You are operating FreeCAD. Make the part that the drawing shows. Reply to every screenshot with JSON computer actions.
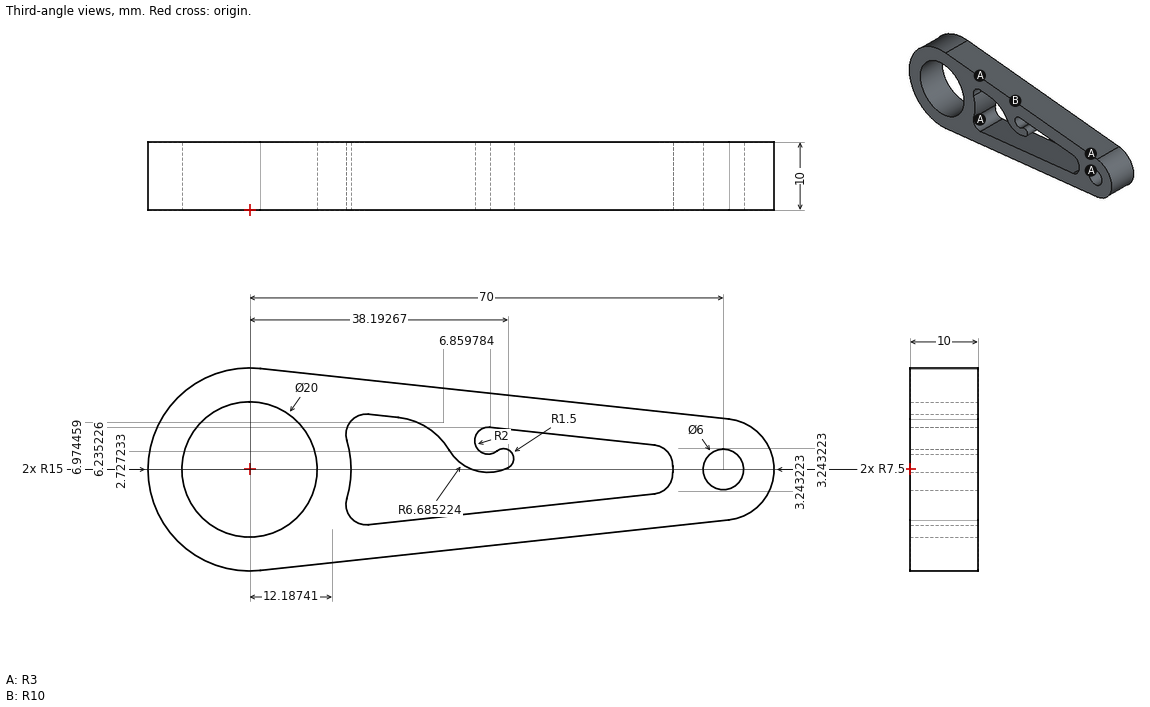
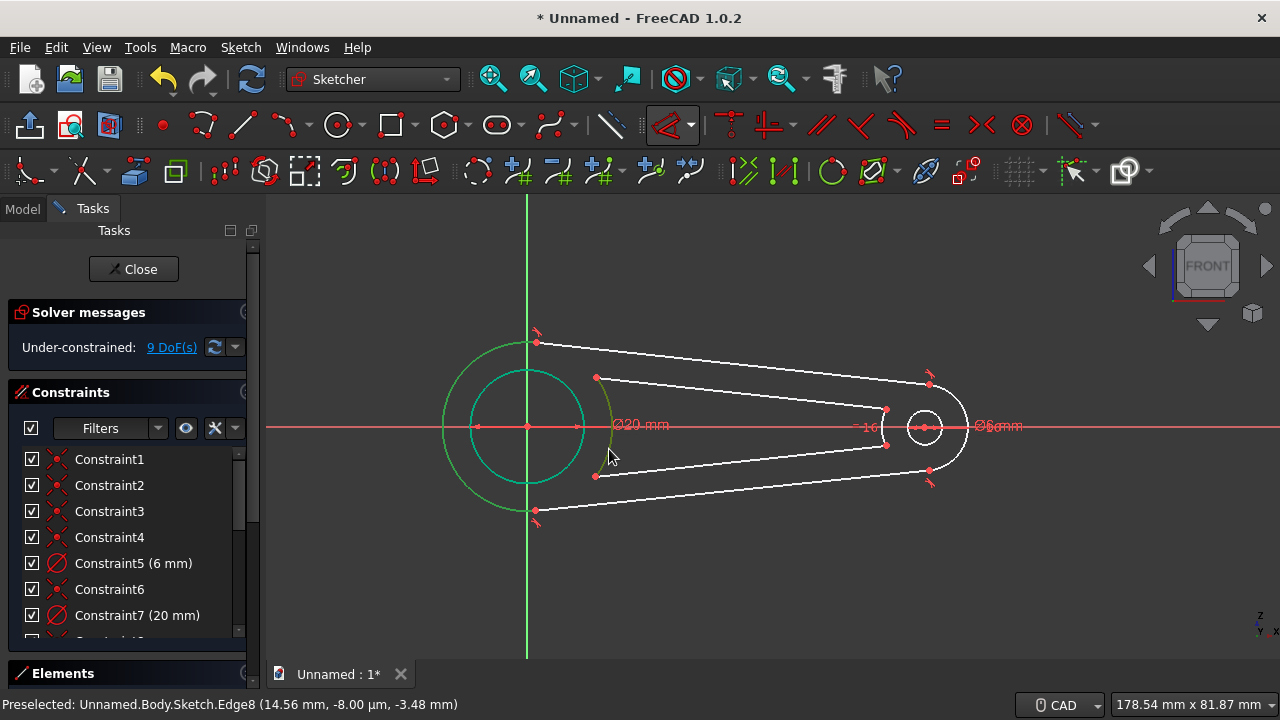
{"action": "left_click", "coordinate": [942, 126]}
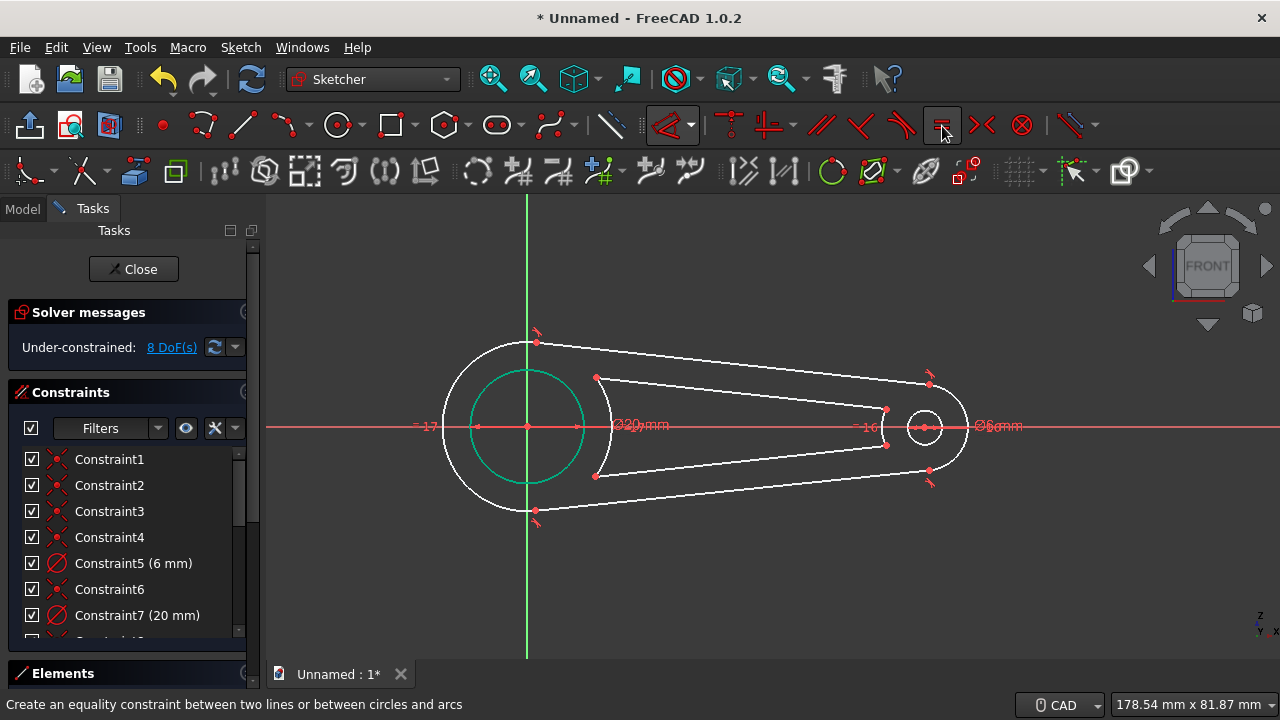
{"action": "left_click", "coordinate": [925, 428]}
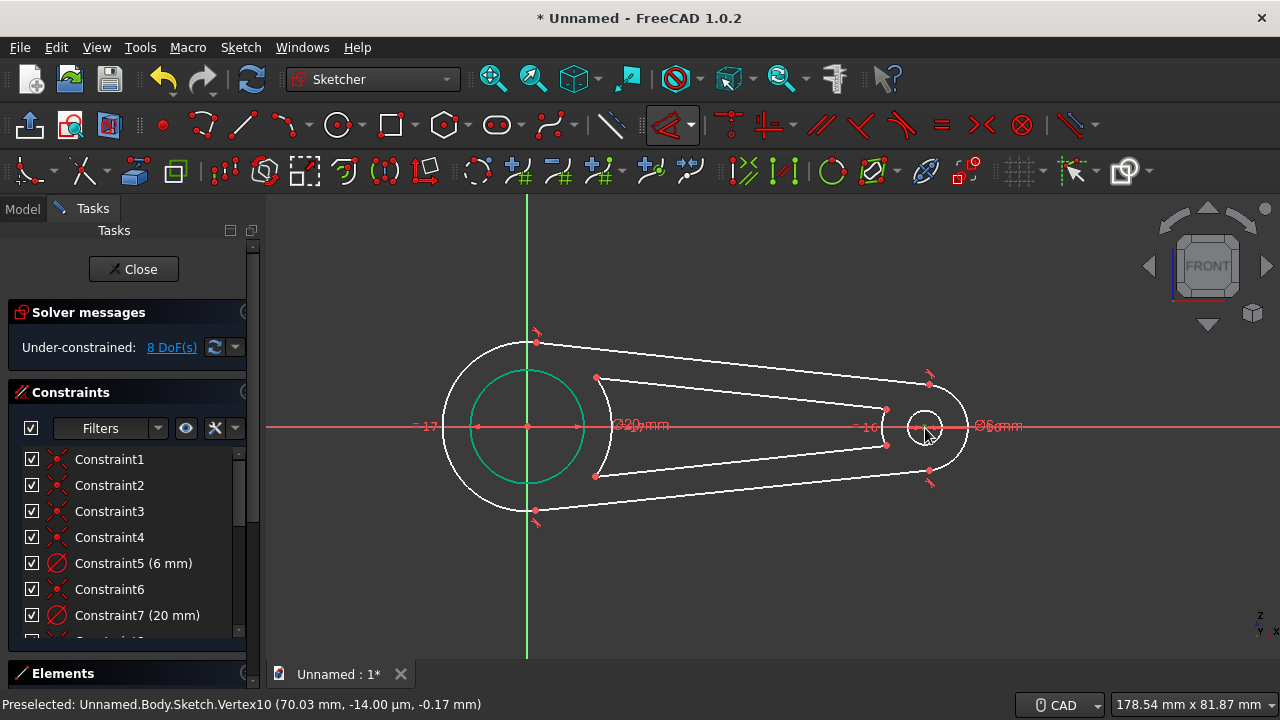
{"action": "left_click", "coordinate": [353, 427]}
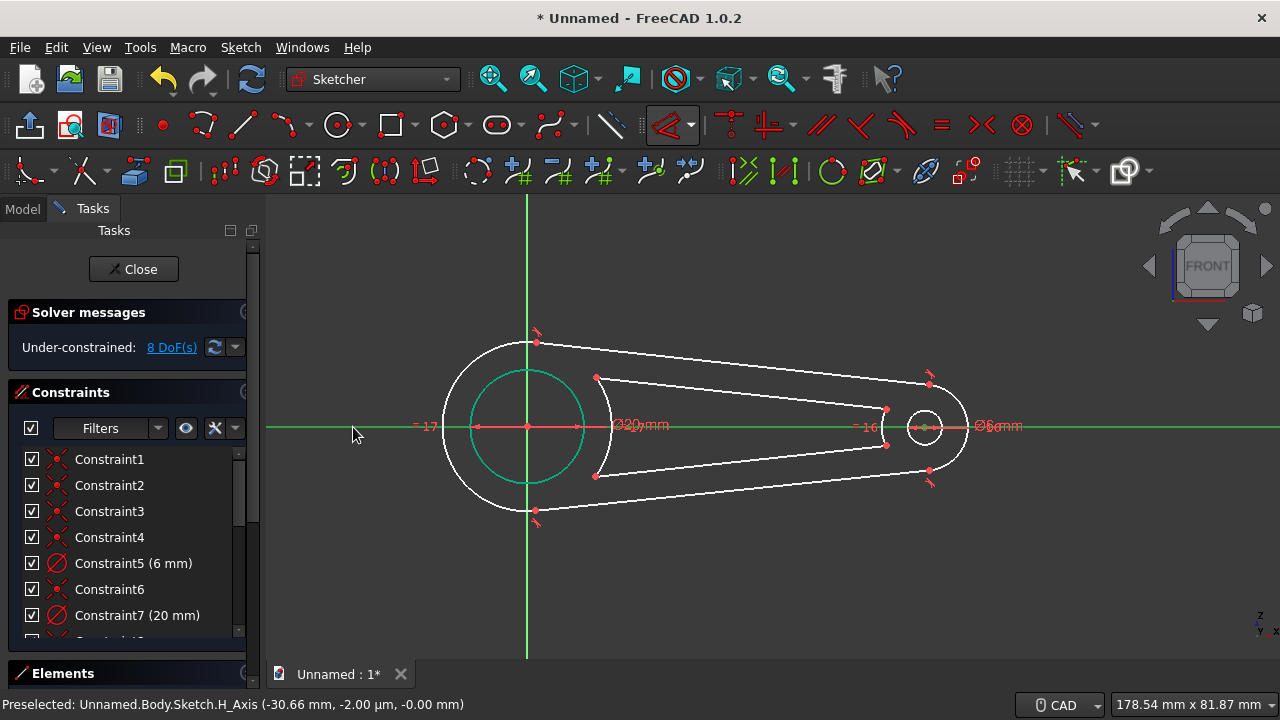
{"action": "left_click", "coordinate": [730, 126]}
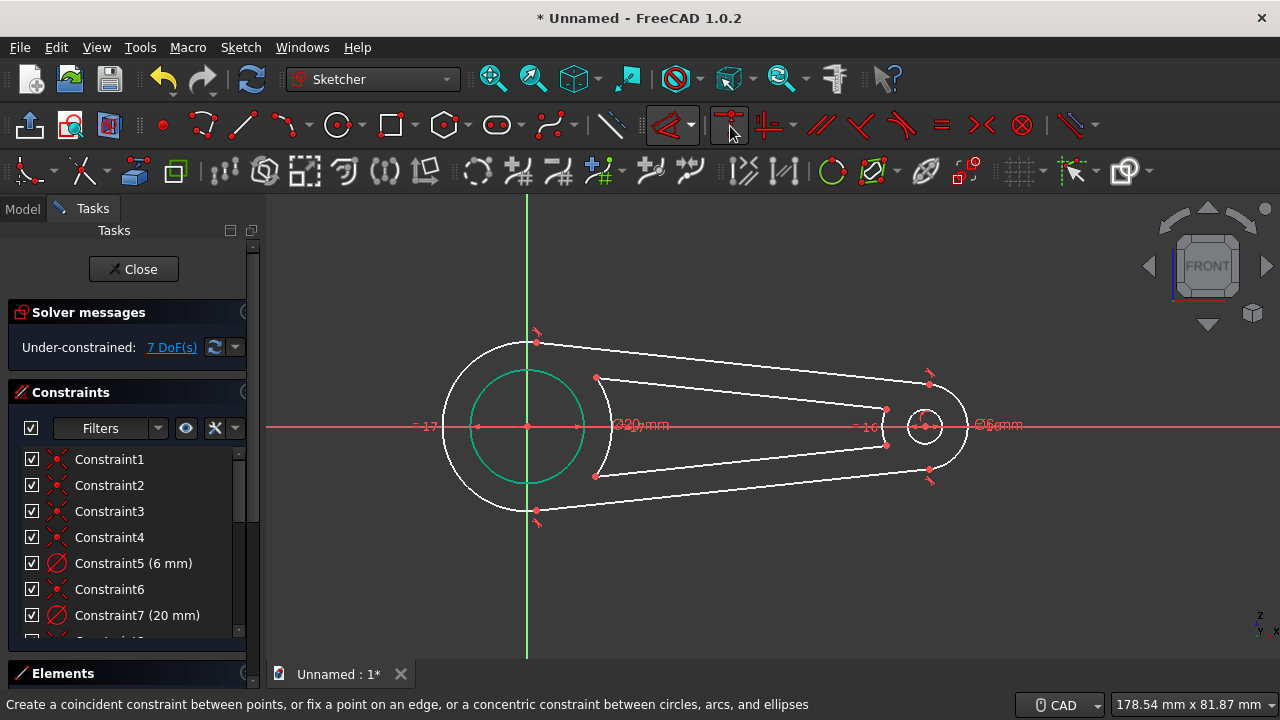
{"action": "left_click", "coordinate": [666, 126]}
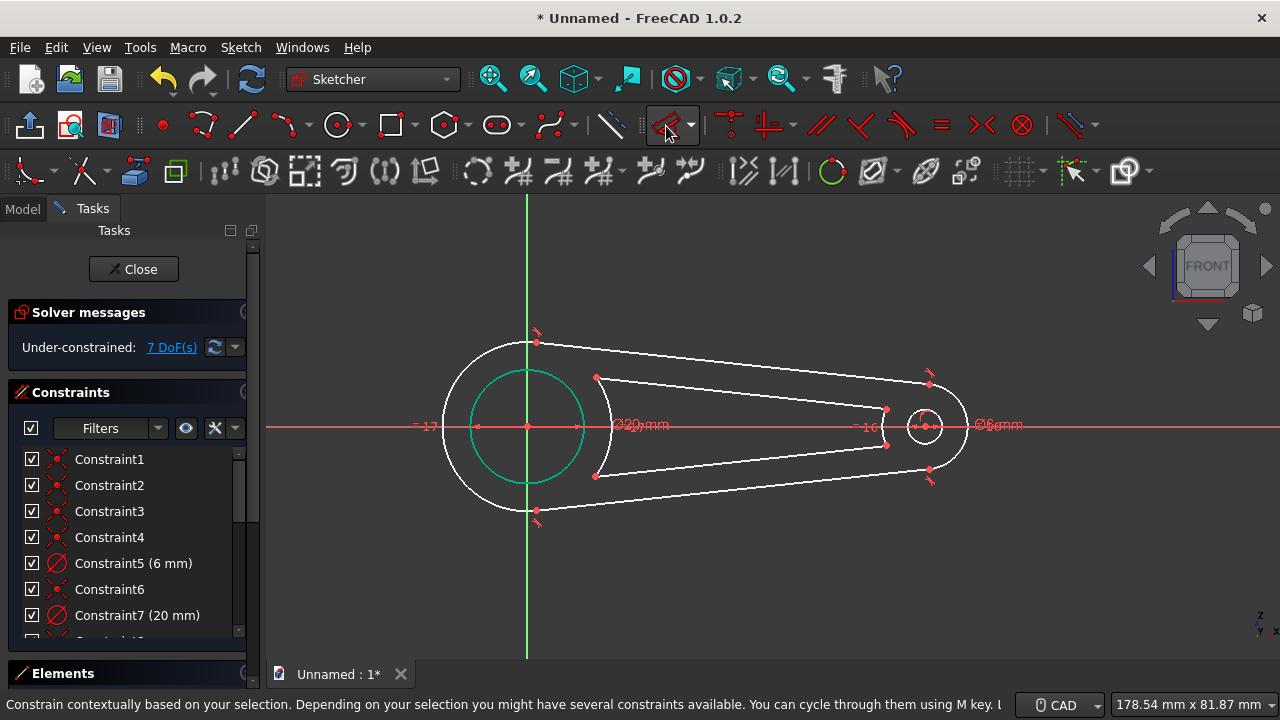
{"action": "left_click", "coordinate": [461, 374]}
{"action": "left_click", "coordinate": [436, 354]}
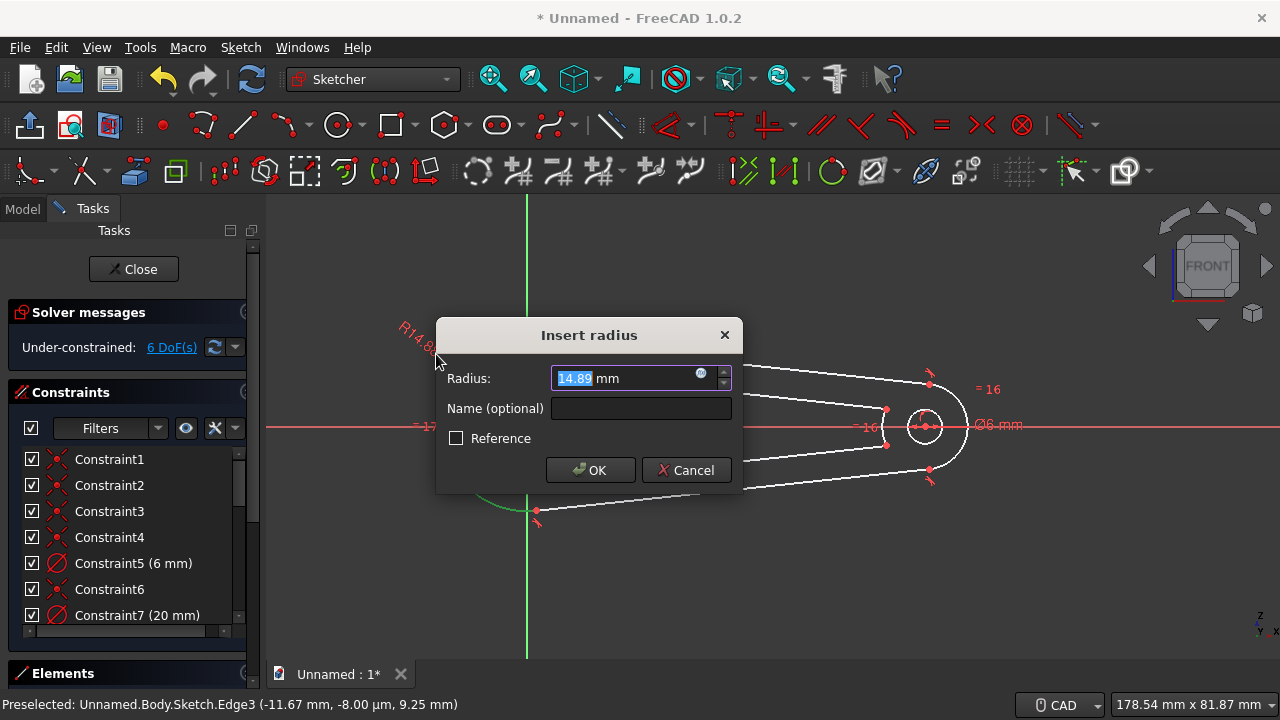
{"action": "type", "text": "15"}
{"action": "key", "text": "Return"}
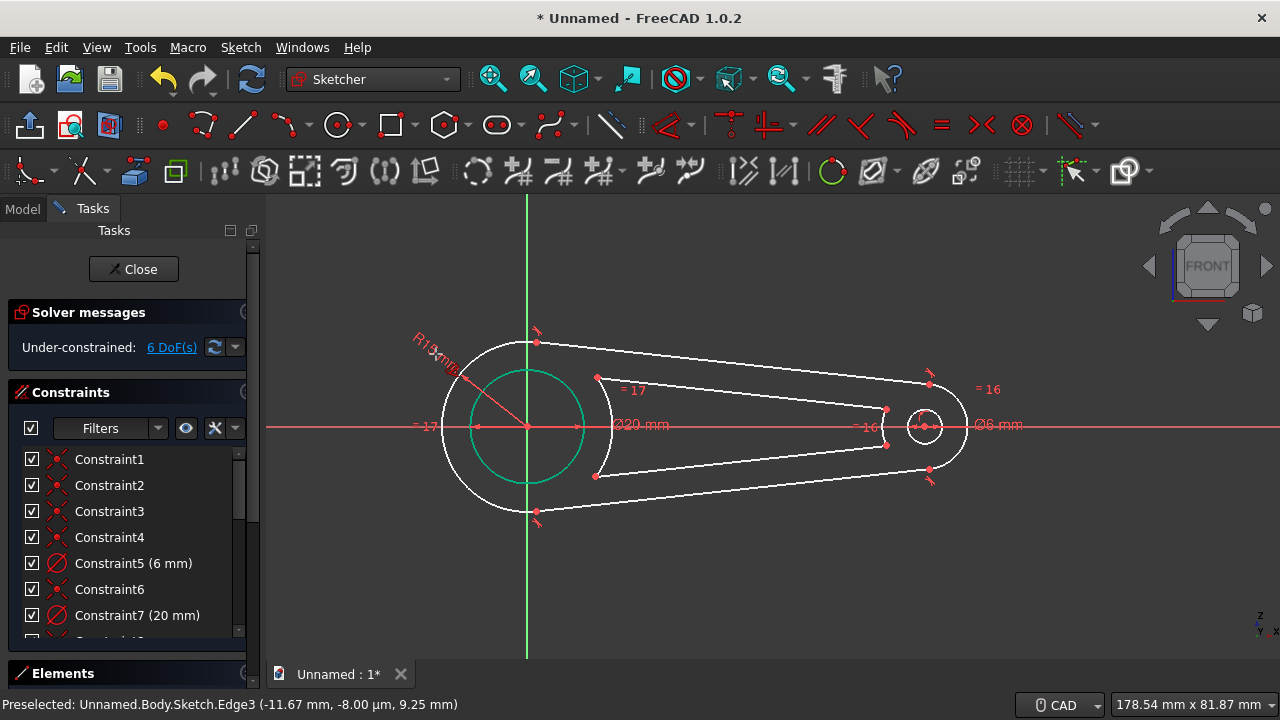
{"action": "left_click", "coordinate": [960, 450]}
{"action": "left_click", "coordinate": [987, 468]}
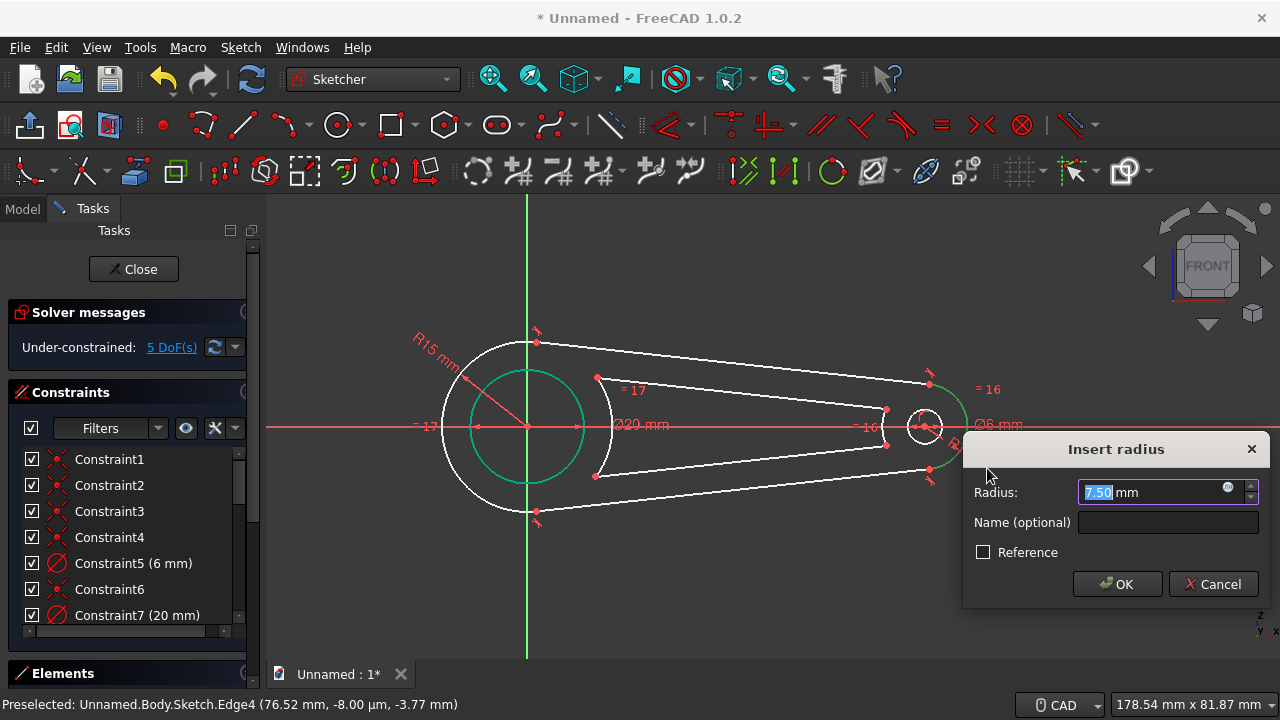
{"action": "type", "text": "7.5"}
{"action": "key", "text": "Return"}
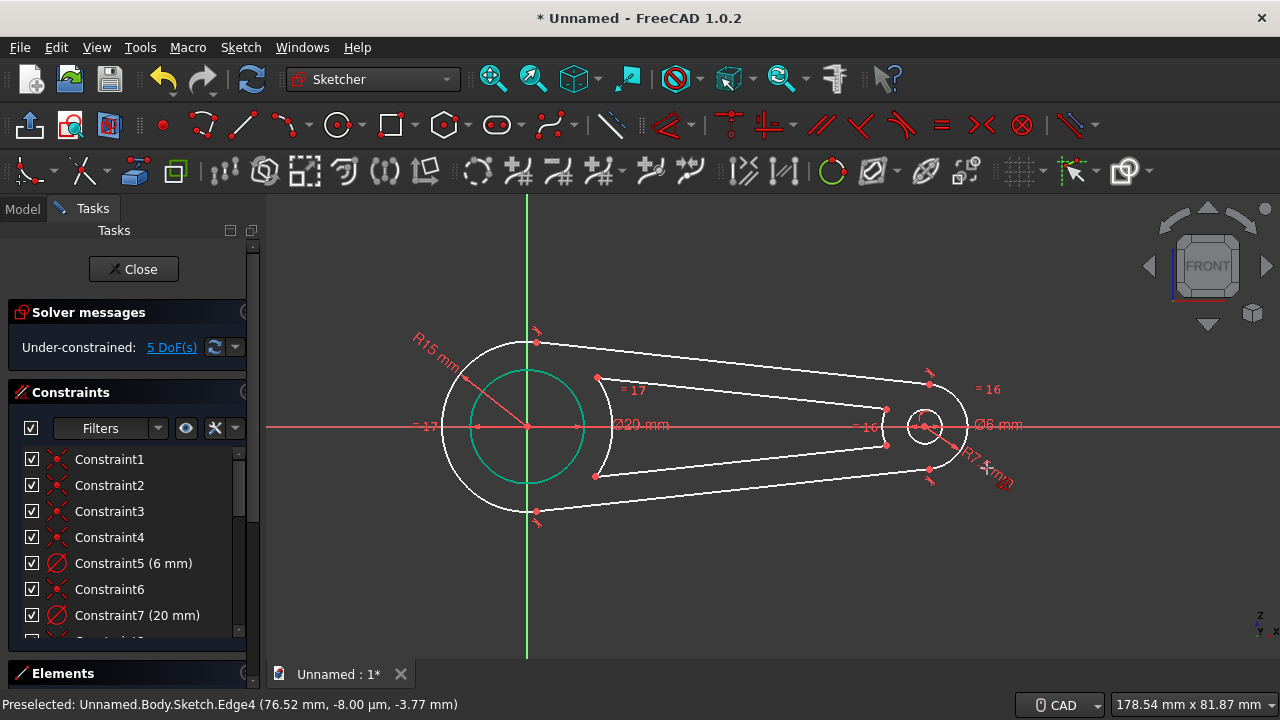
{"action": "left_click", "coordinate": [925, 427]}
{"action": "left_click", "coordinate": [865, 393]}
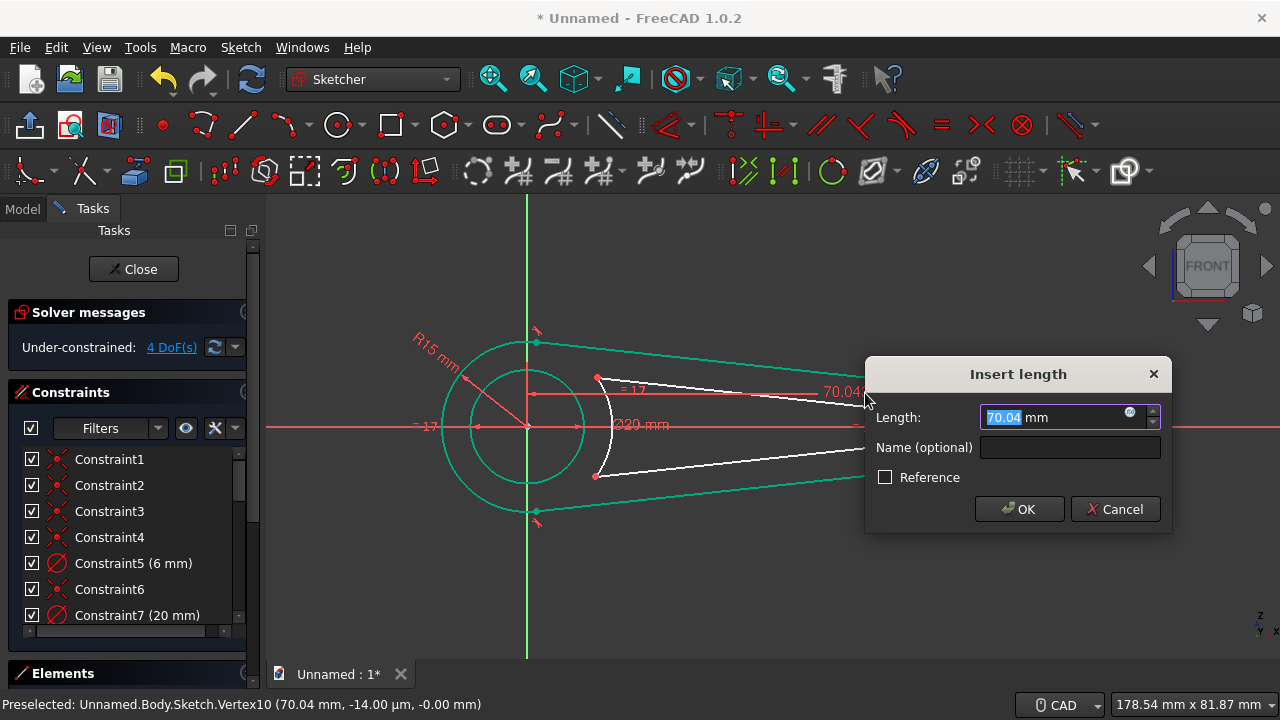
{"action": "type", "text": "70"}
{"action": "key", "text": "Return"}